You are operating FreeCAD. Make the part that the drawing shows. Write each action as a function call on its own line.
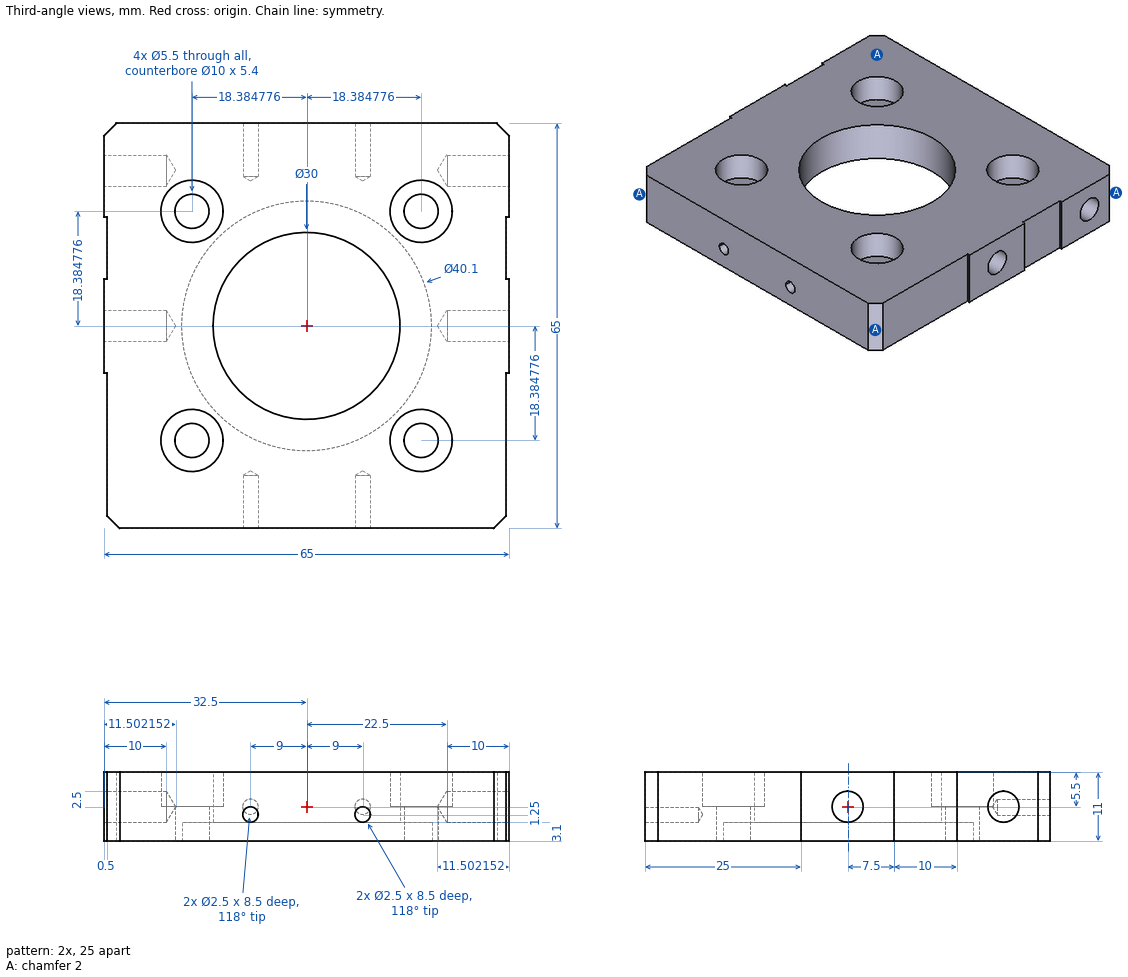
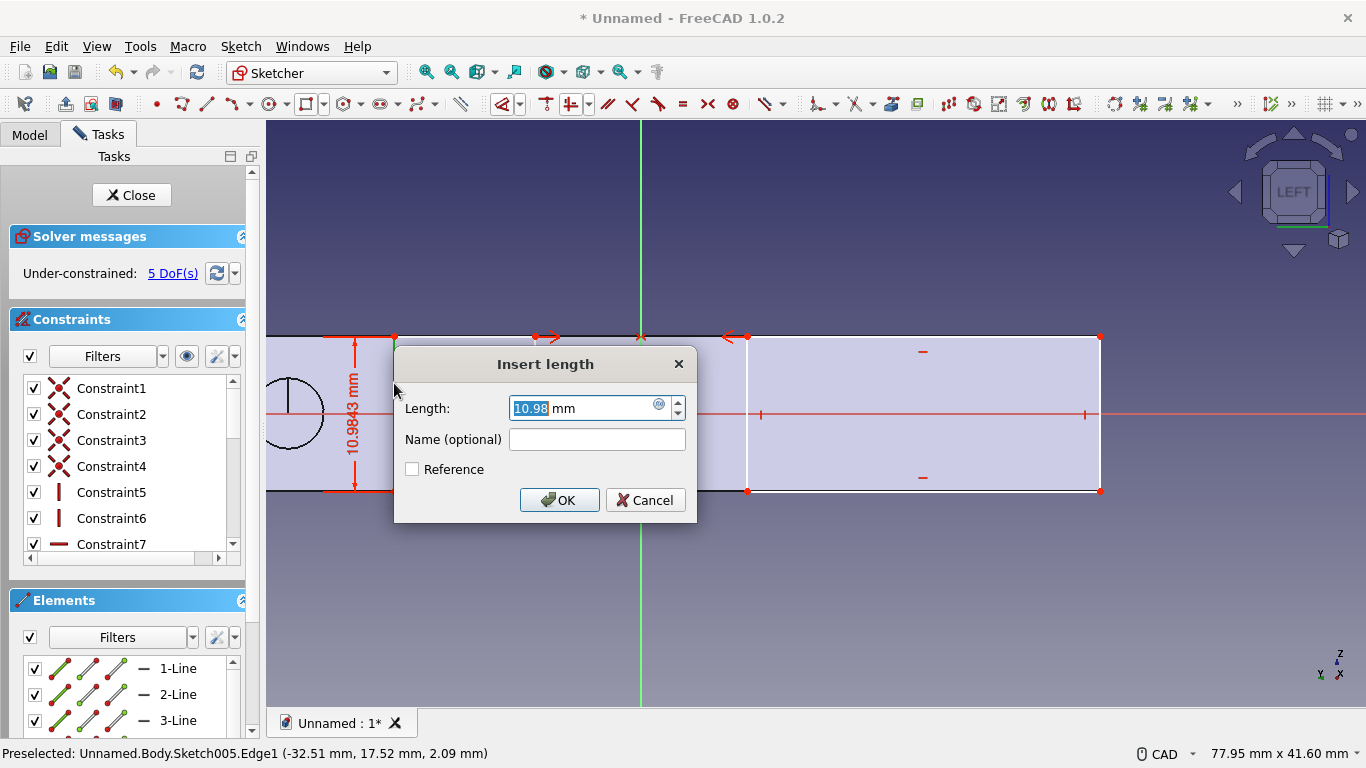
text(11)
key(Return)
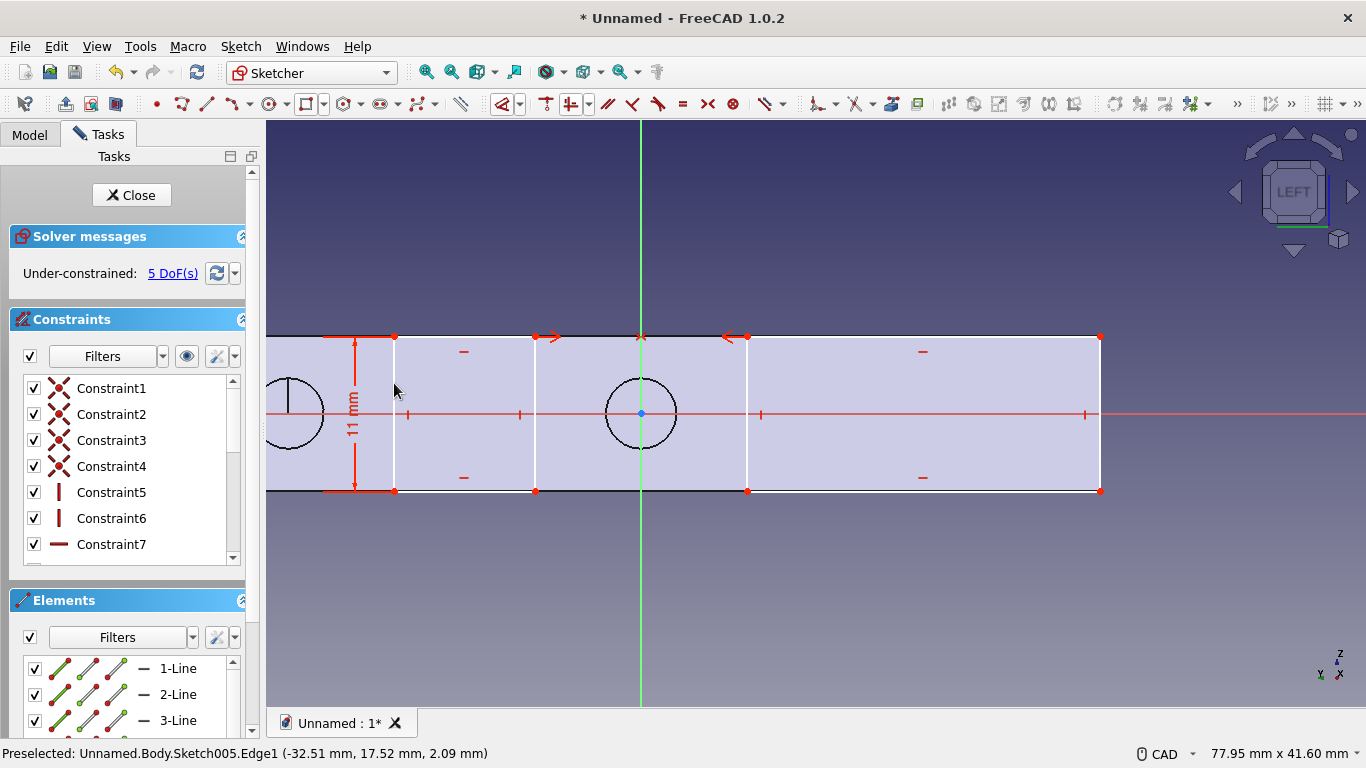
click(436, 492)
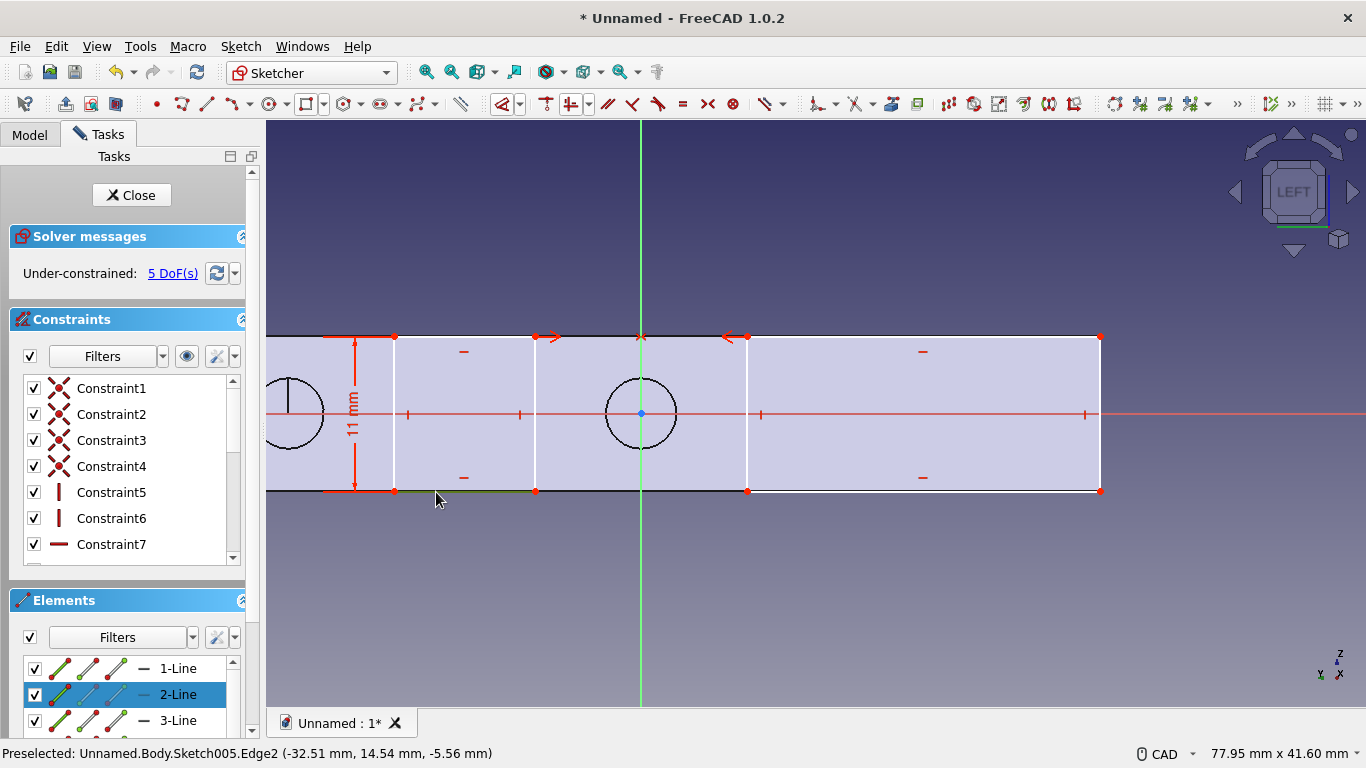
key(l)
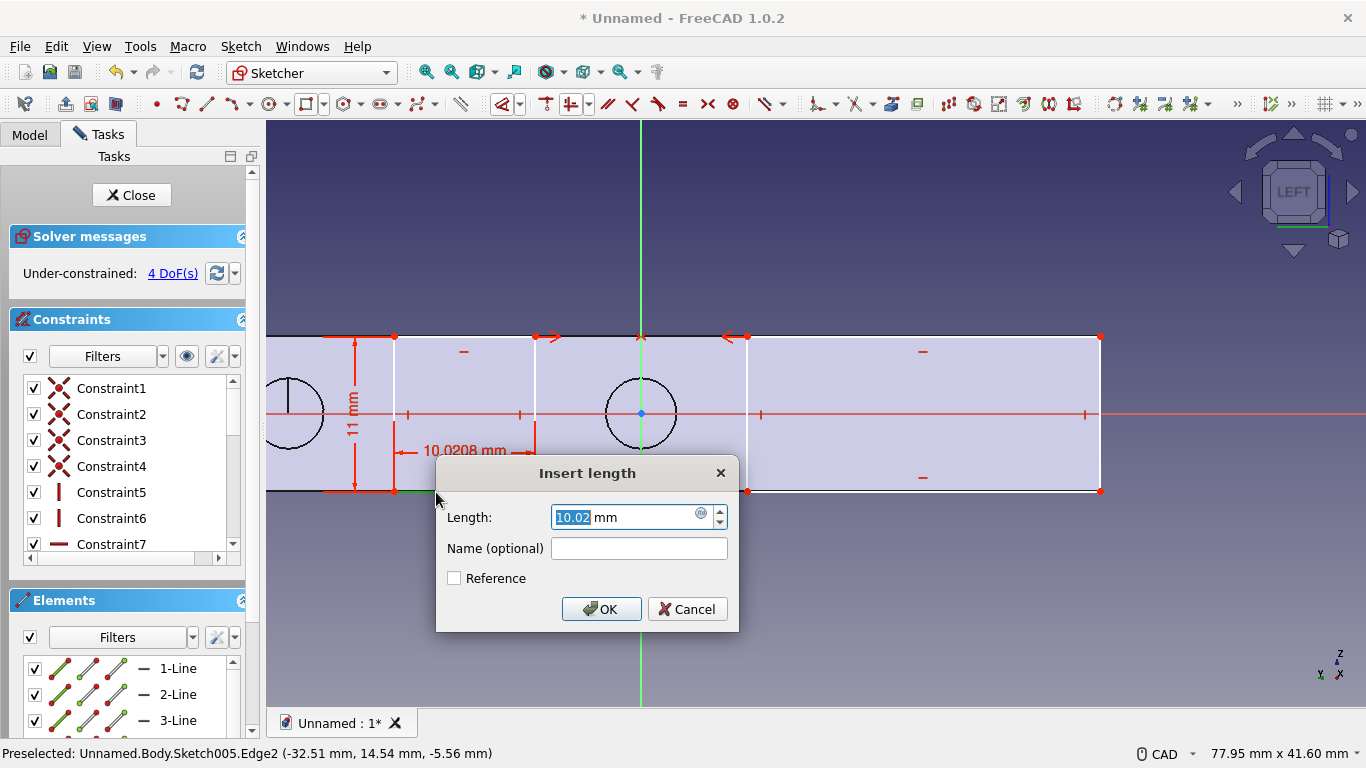
text(10)
key(Return)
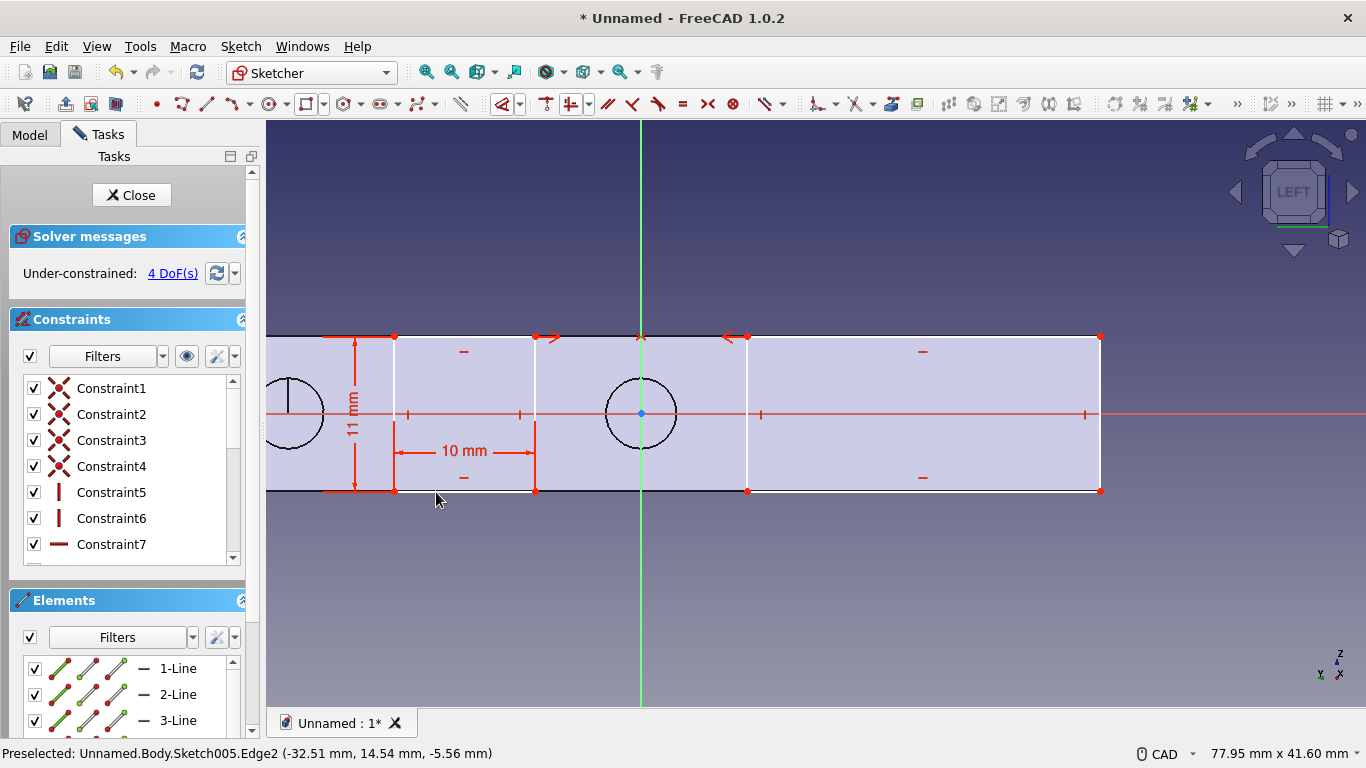
click(747, 383)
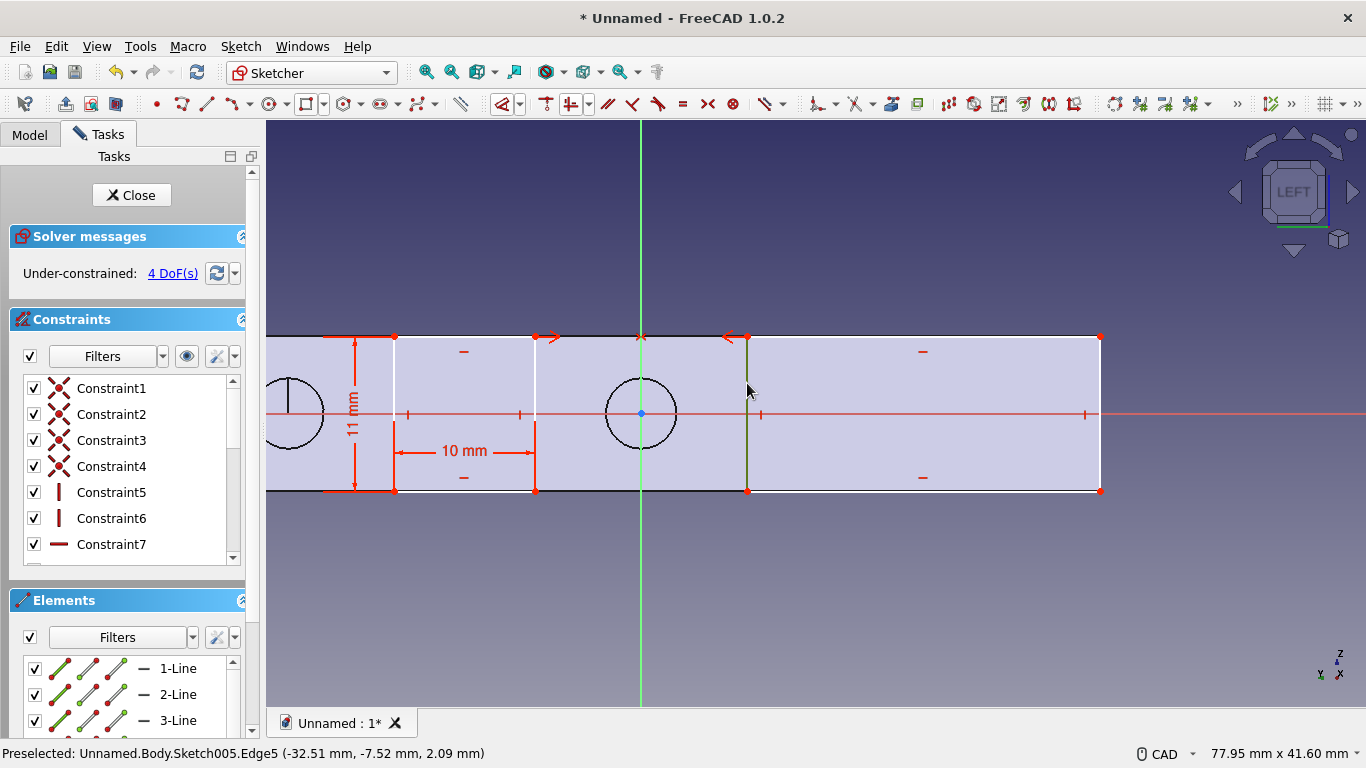
key(i)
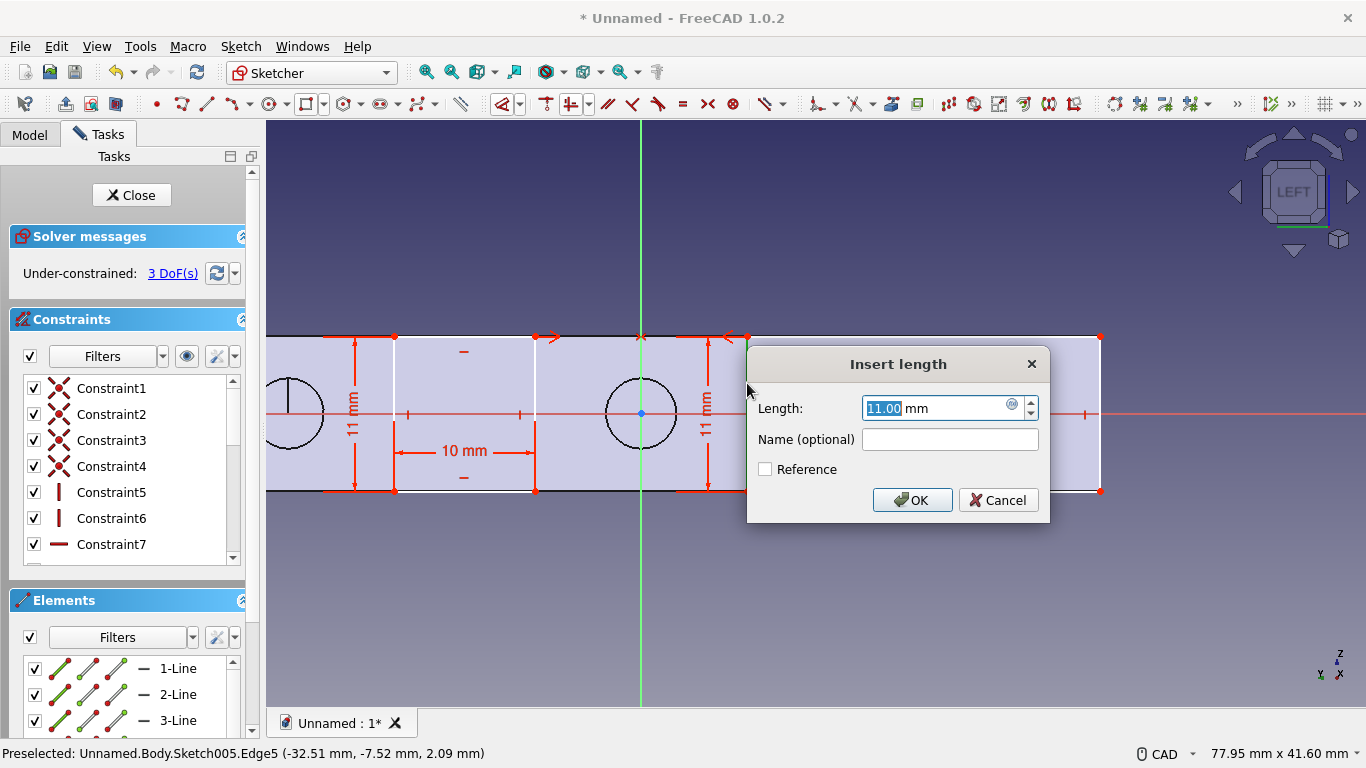
text(11)
key(Return)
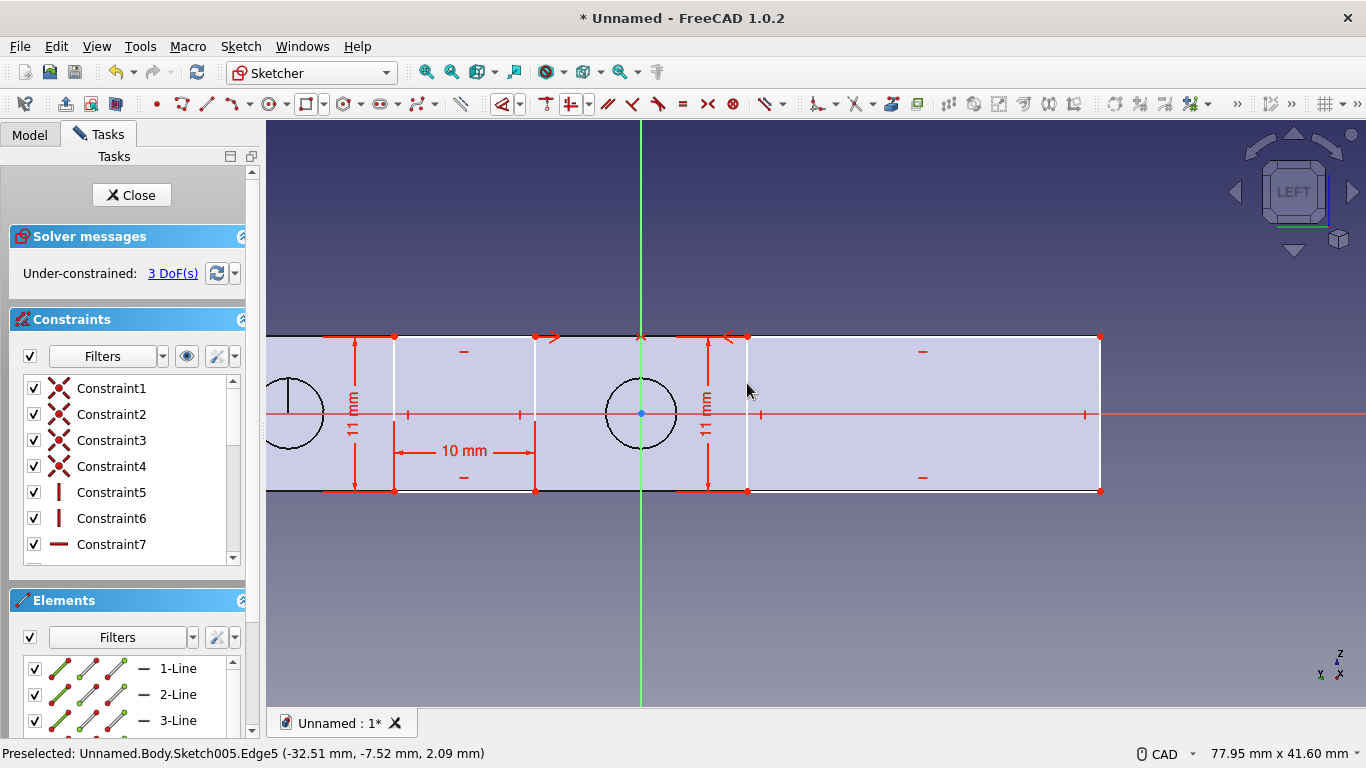
click(853, 492)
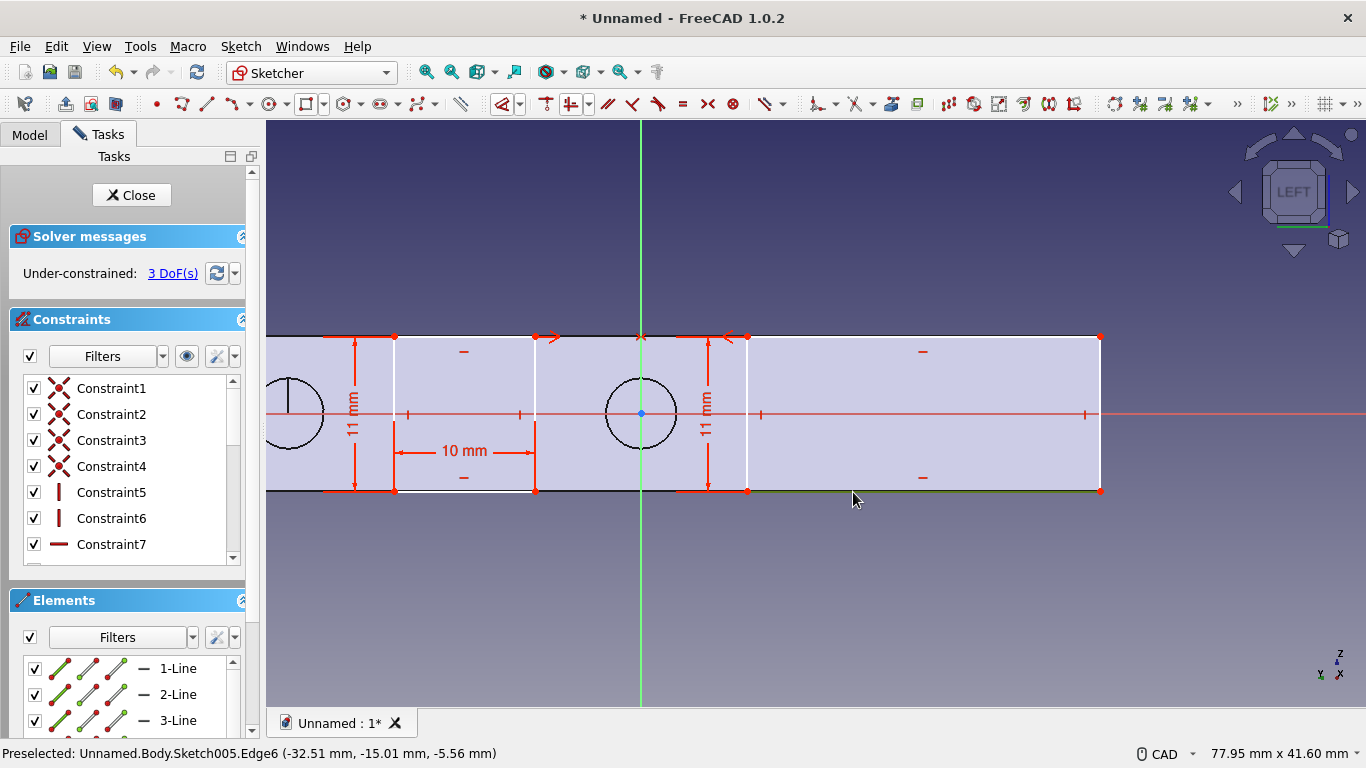
click(520, 104)